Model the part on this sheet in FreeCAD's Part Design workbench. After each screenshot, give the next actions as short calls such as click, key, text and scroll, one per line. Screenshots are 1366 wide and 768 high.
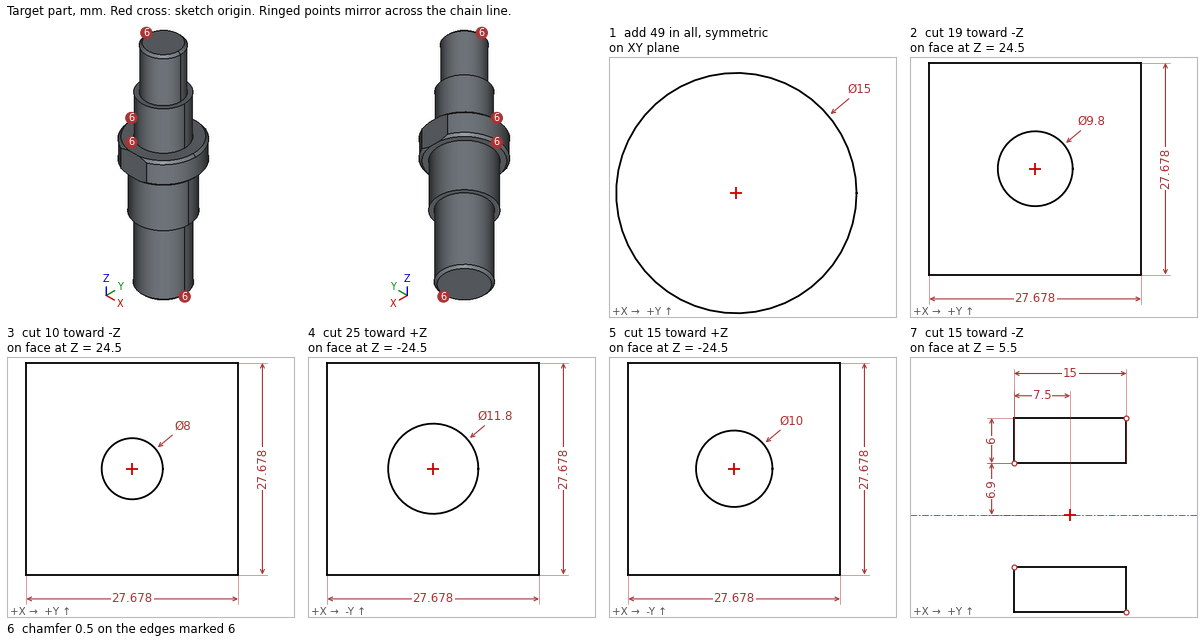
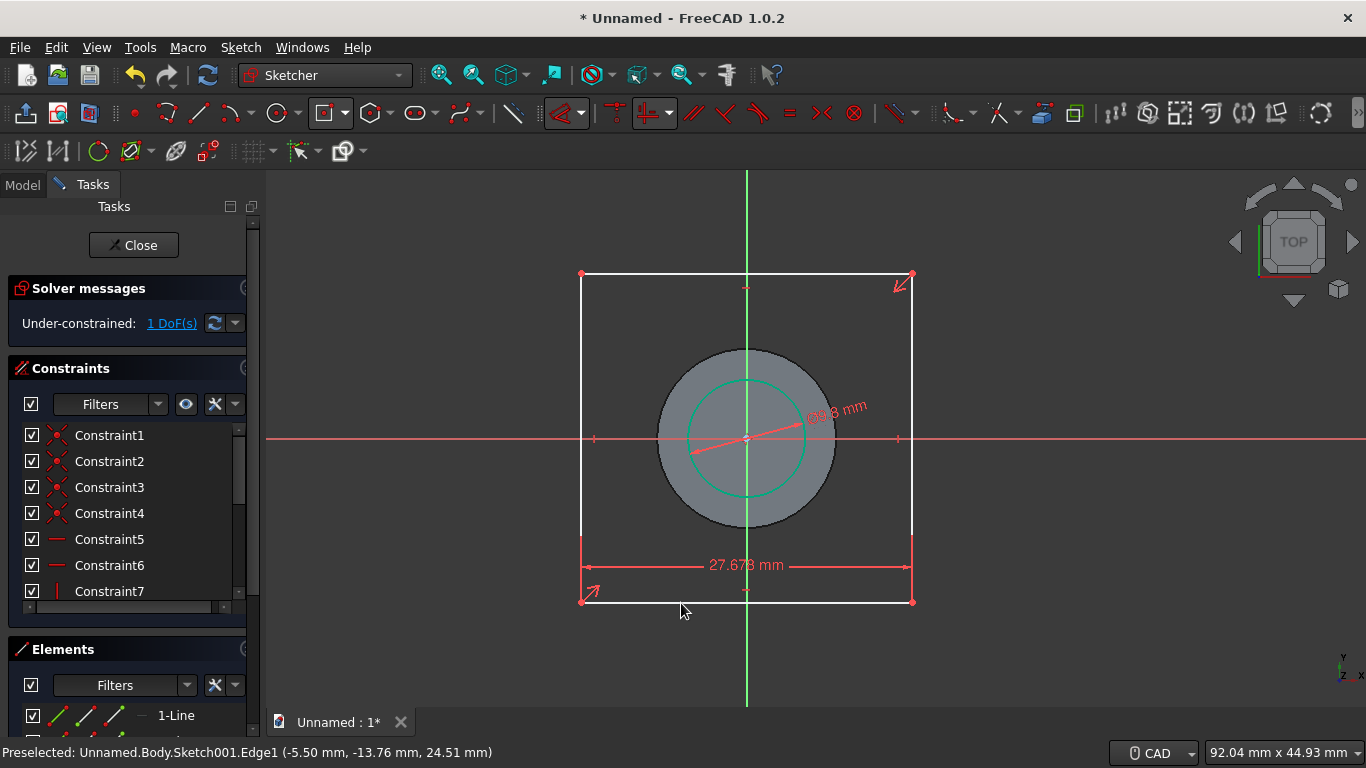
click(912, 504)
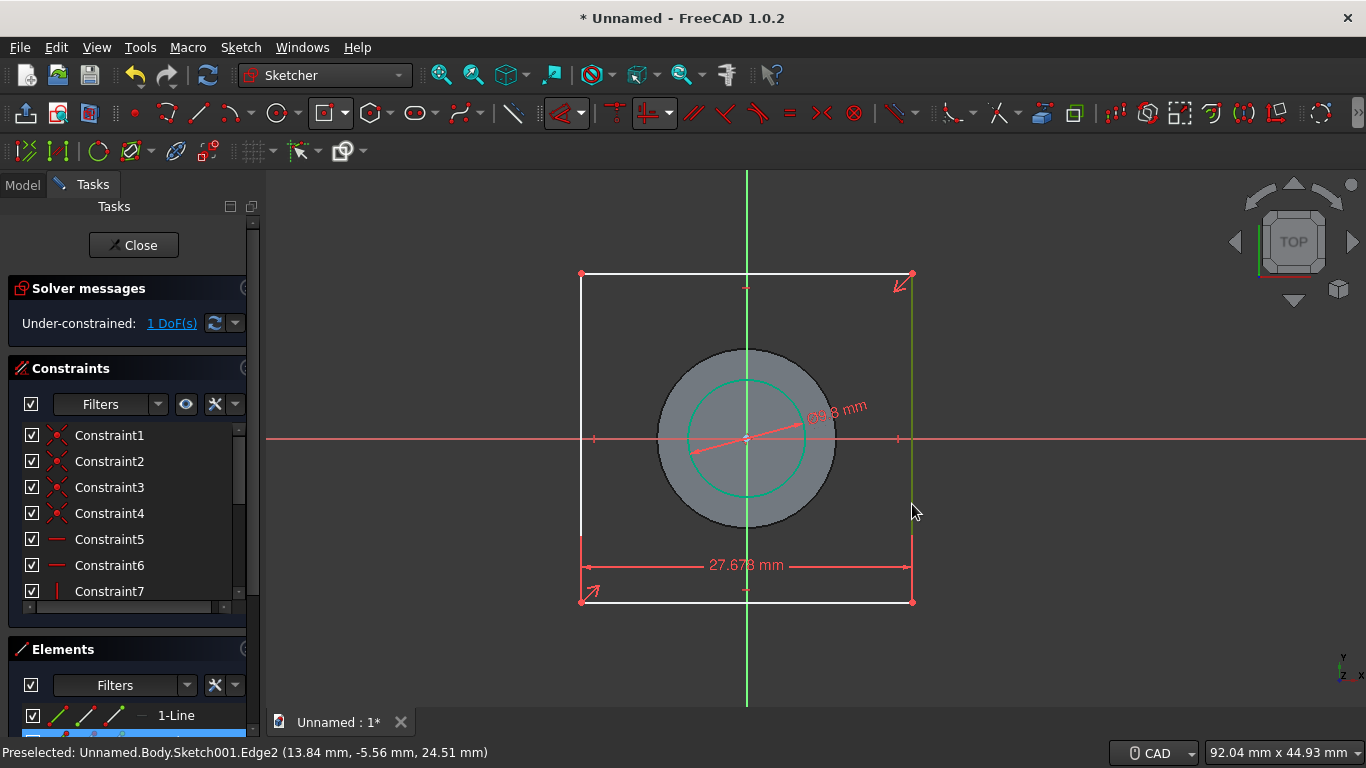
click(584, 114)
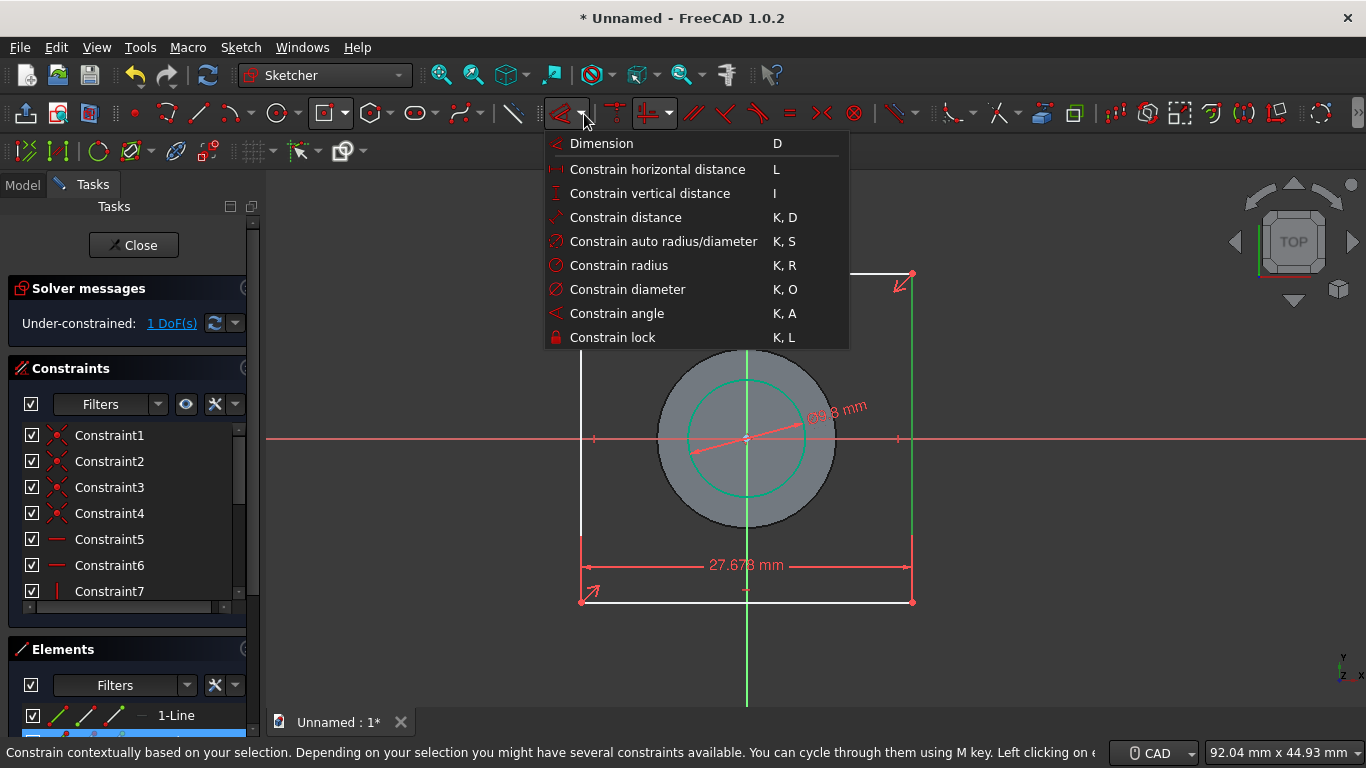
click(697, 193)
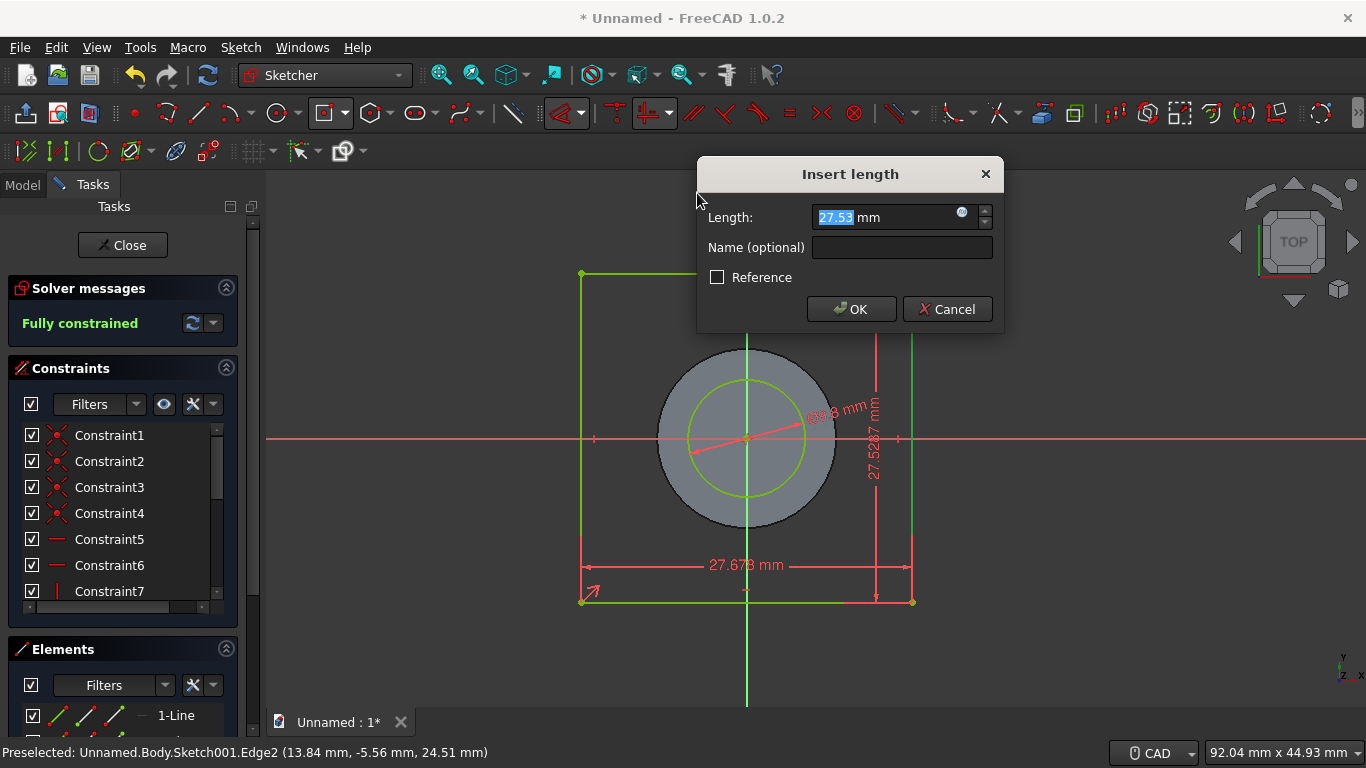
text(27.678)
key(Return)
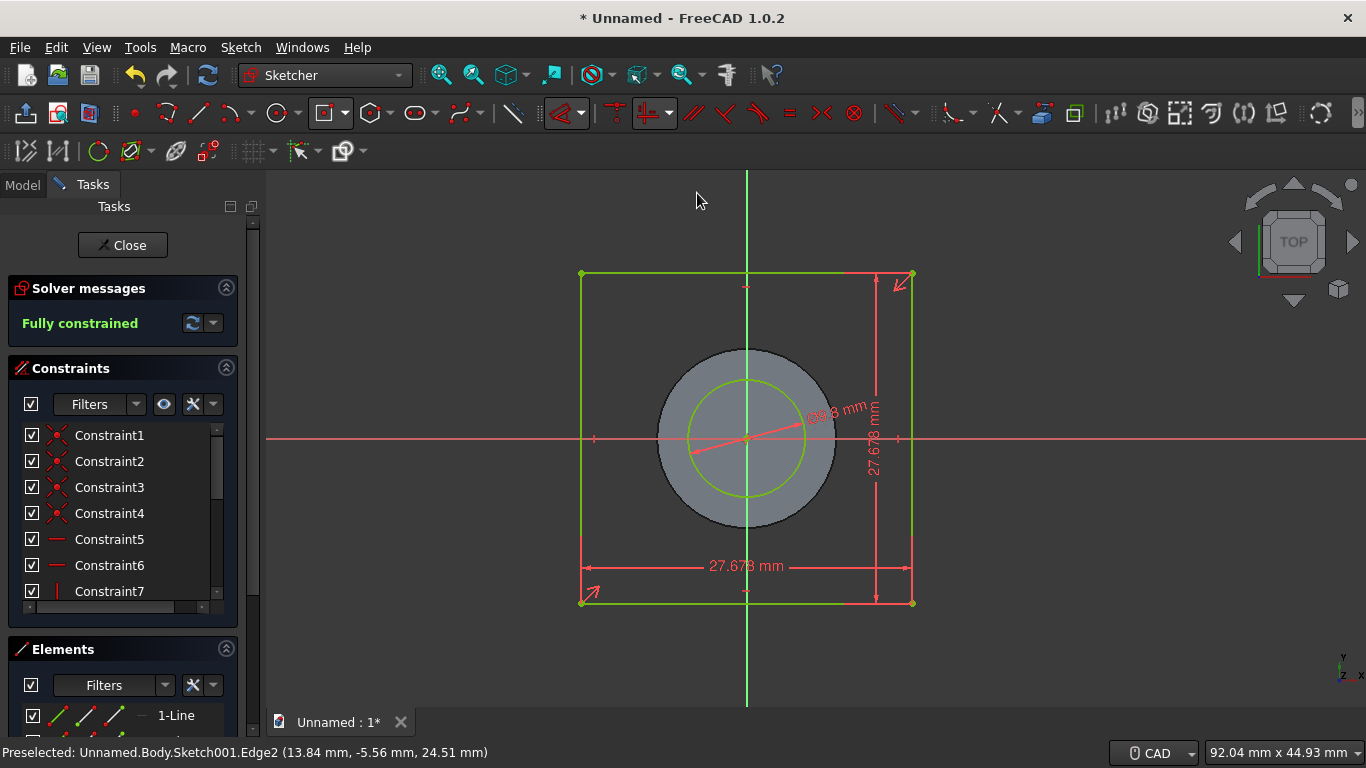
click(123, 245)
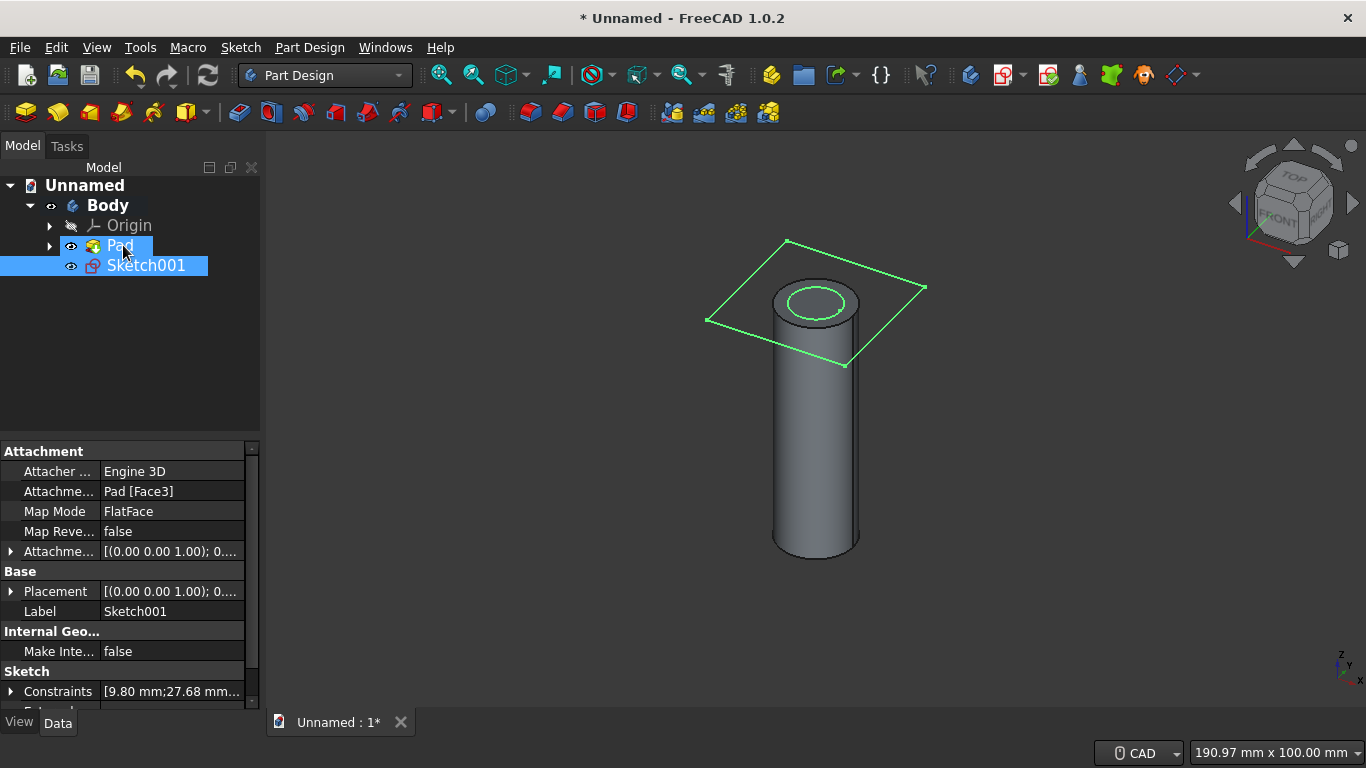
click(240, 112)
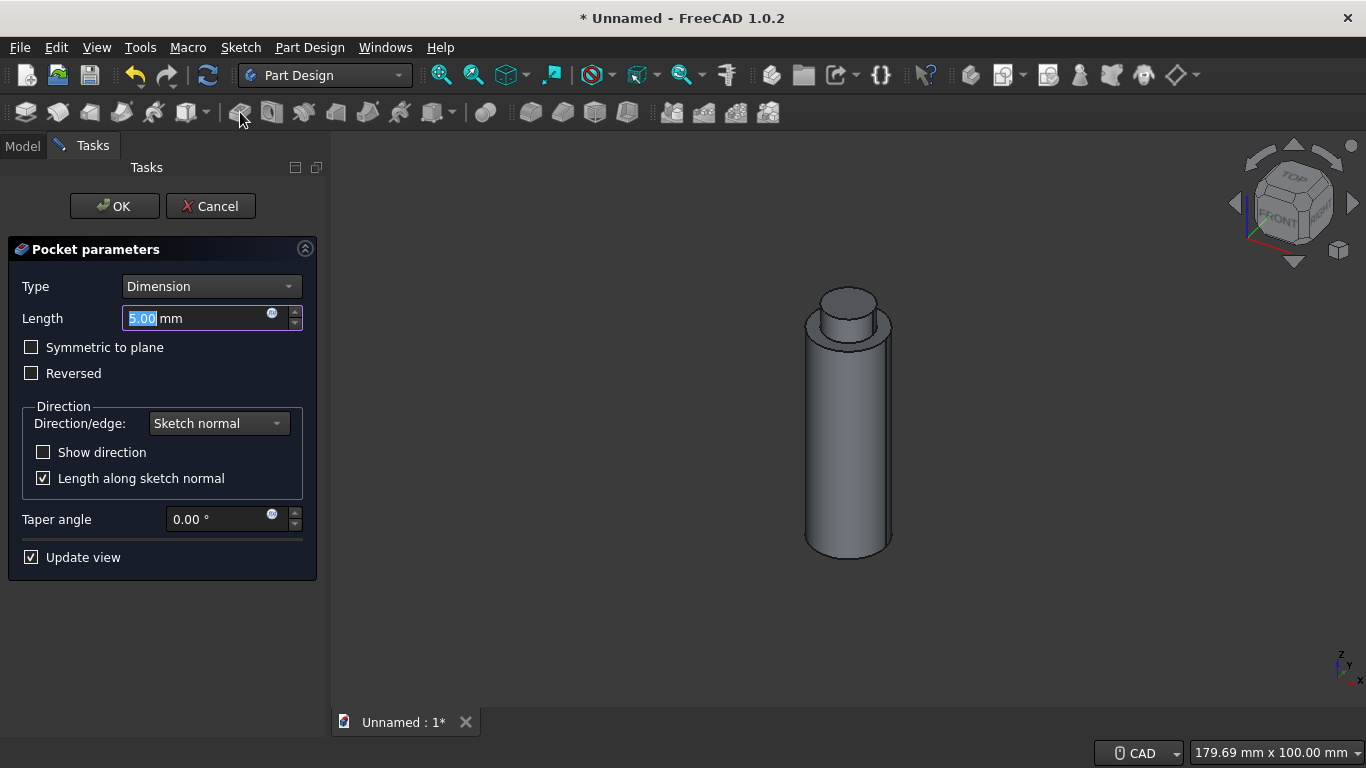
text(19)
key(Tab)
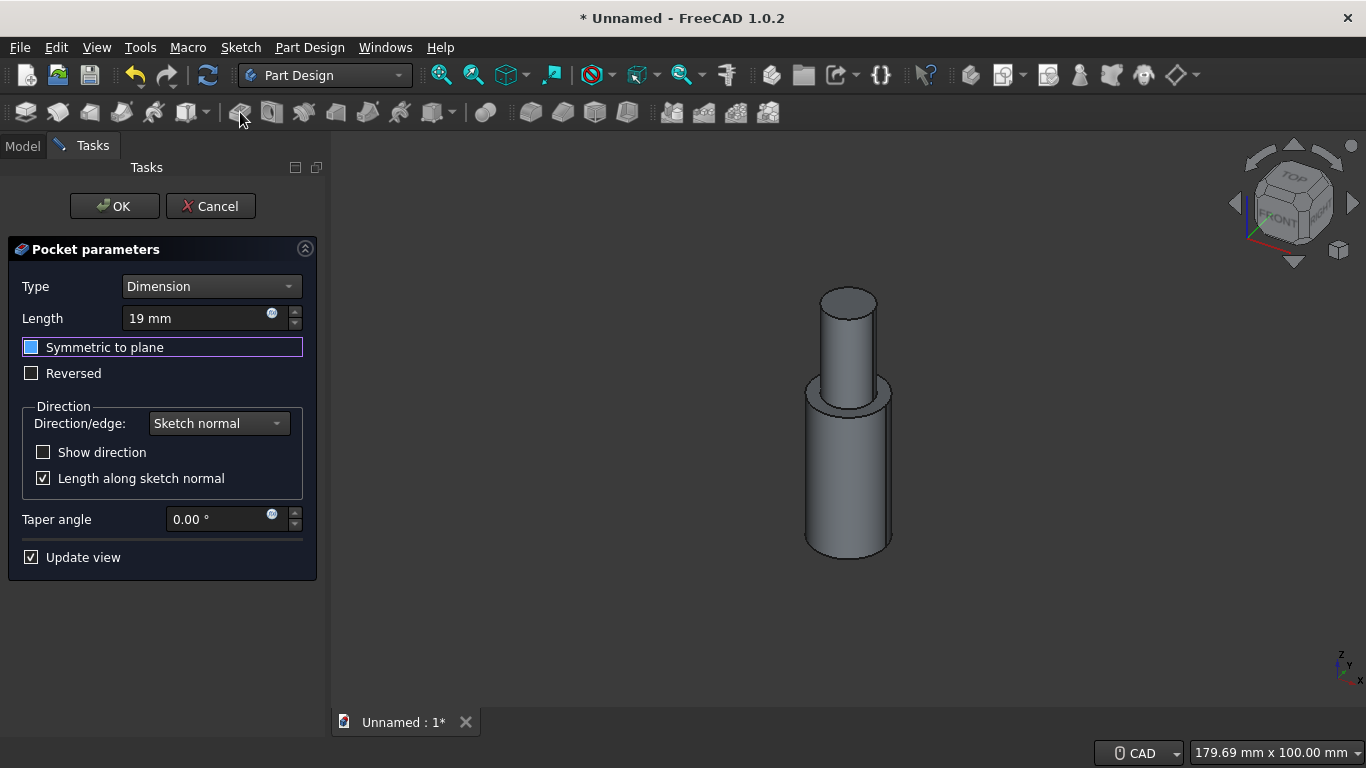
click(115, 206)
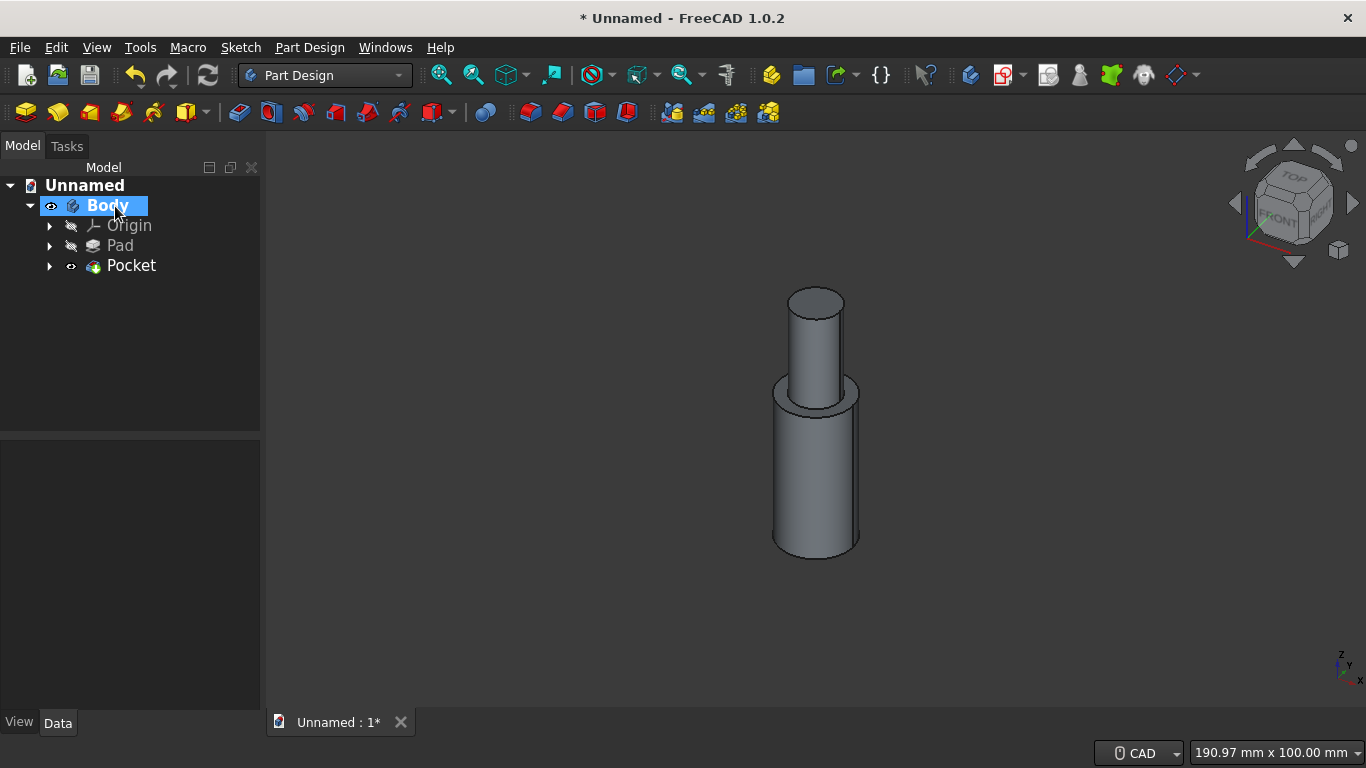
click(816, 302)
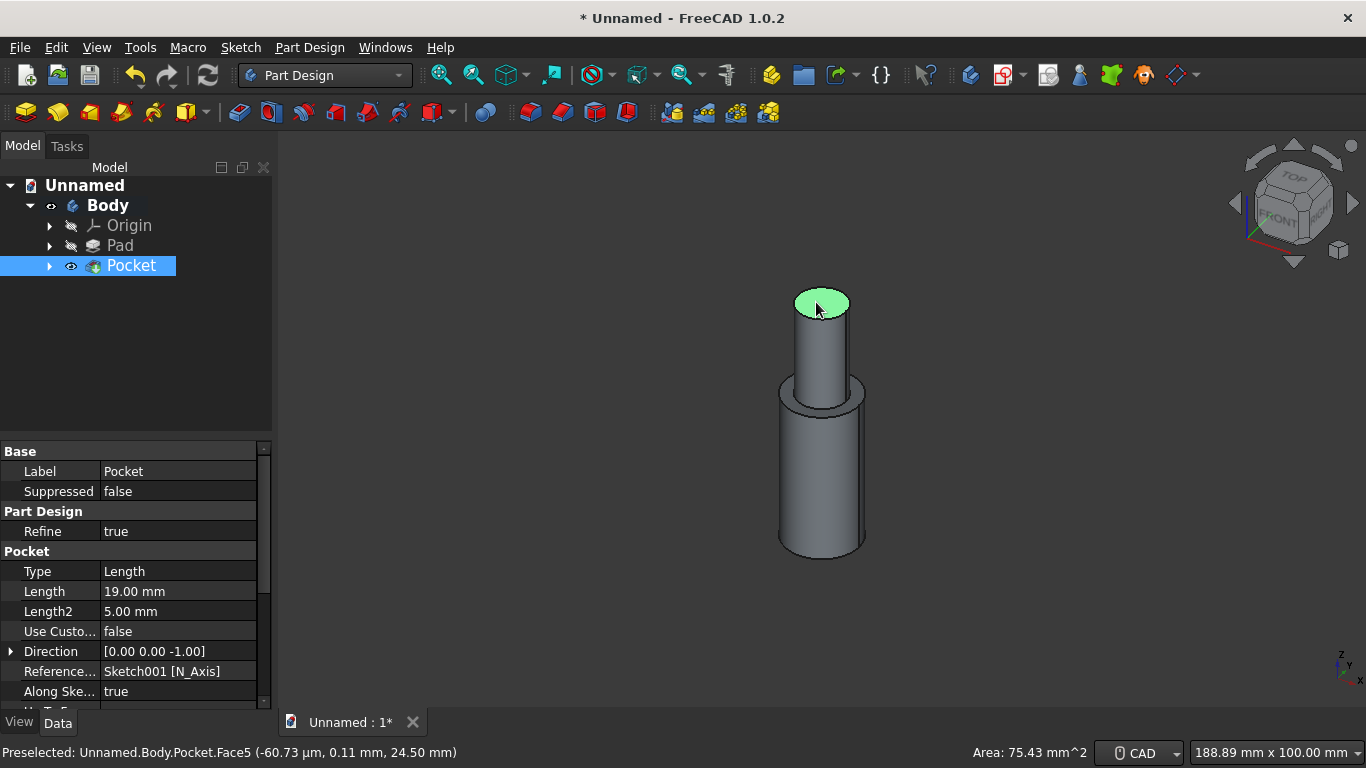
click(1004, 76)